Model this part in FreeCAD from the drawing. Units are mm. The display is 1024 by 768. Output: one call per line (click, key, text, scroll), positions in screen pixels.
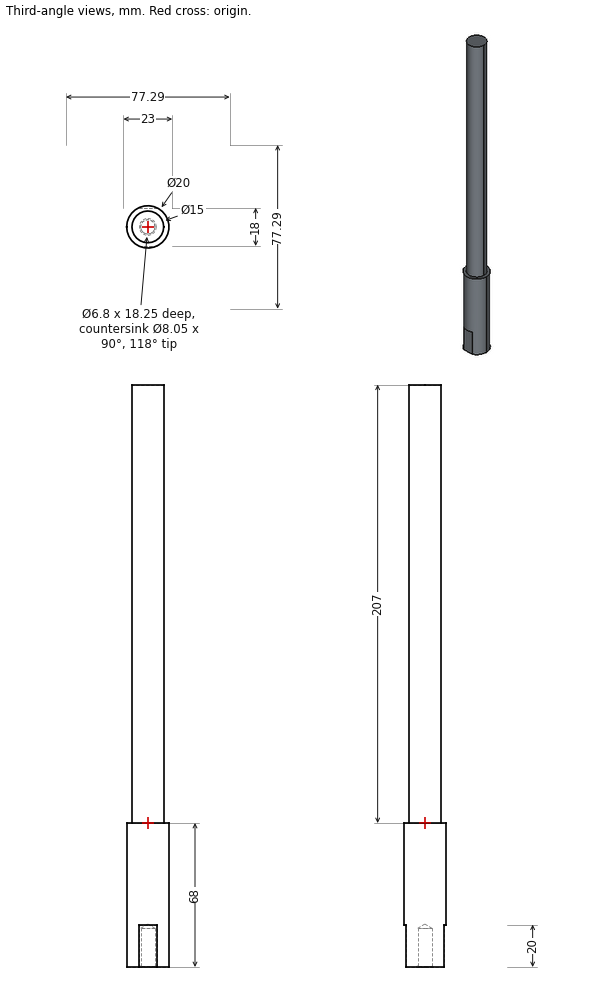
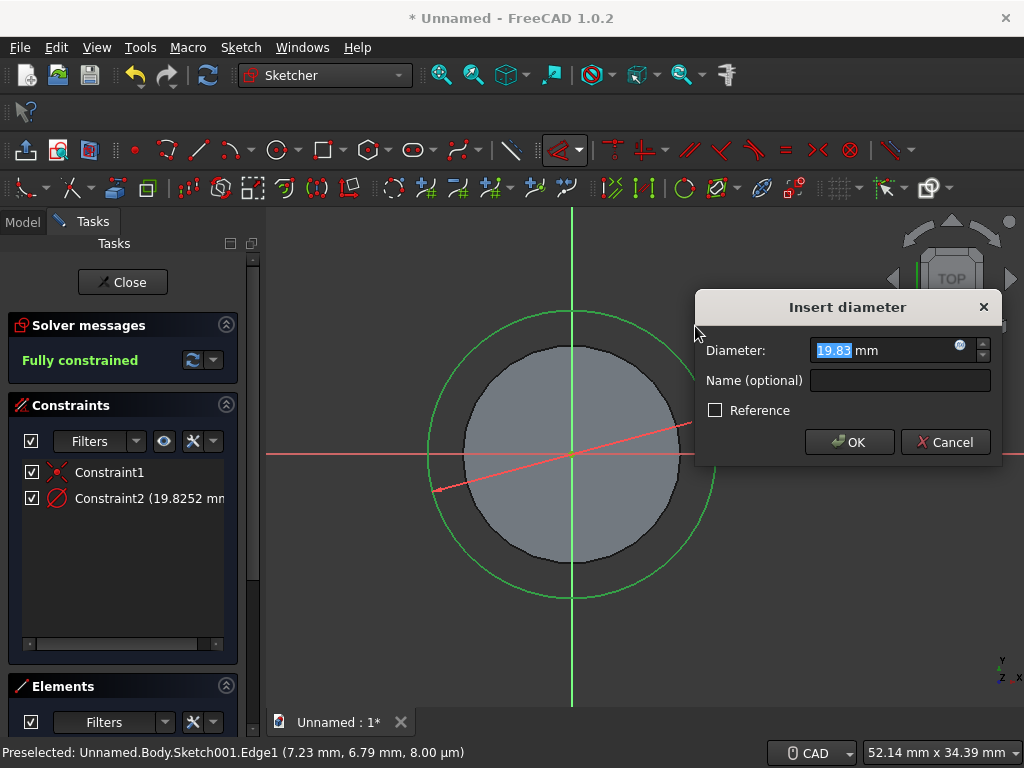
text(20)
key(Return)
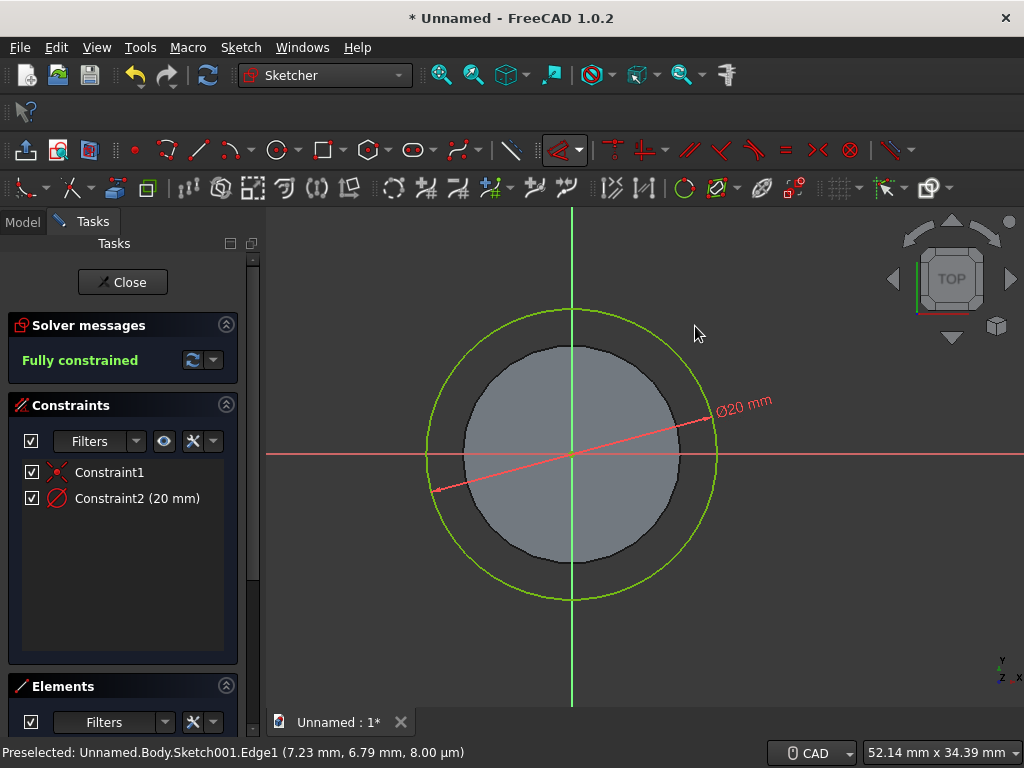
click(123, 282)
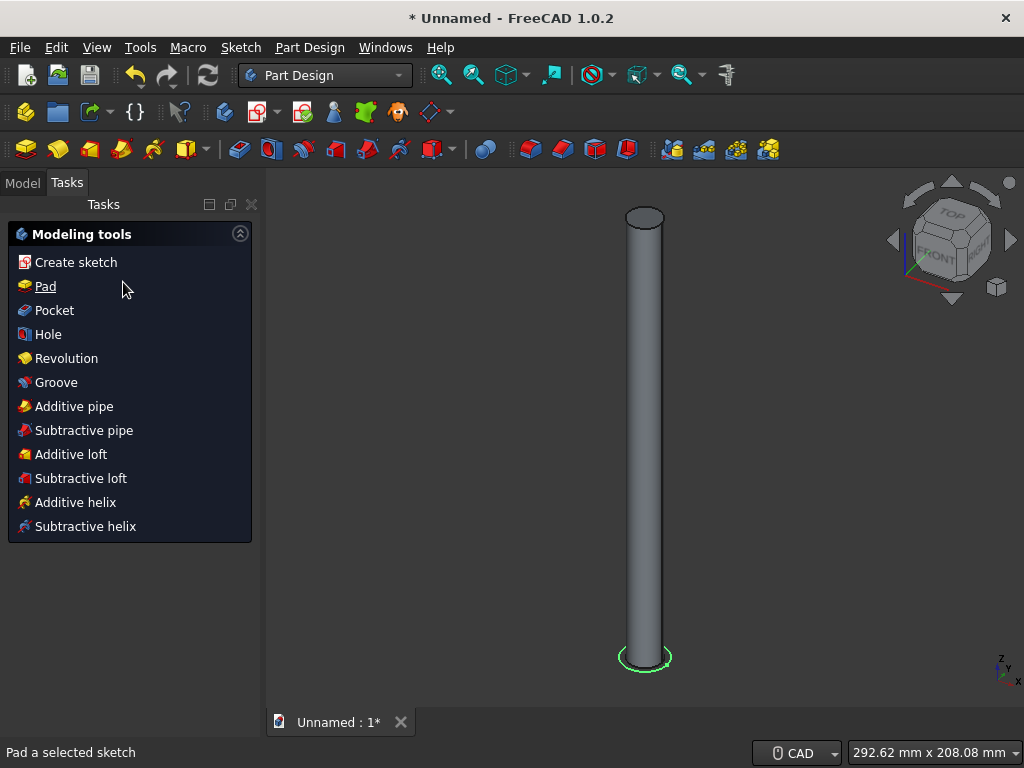
click(26, 150)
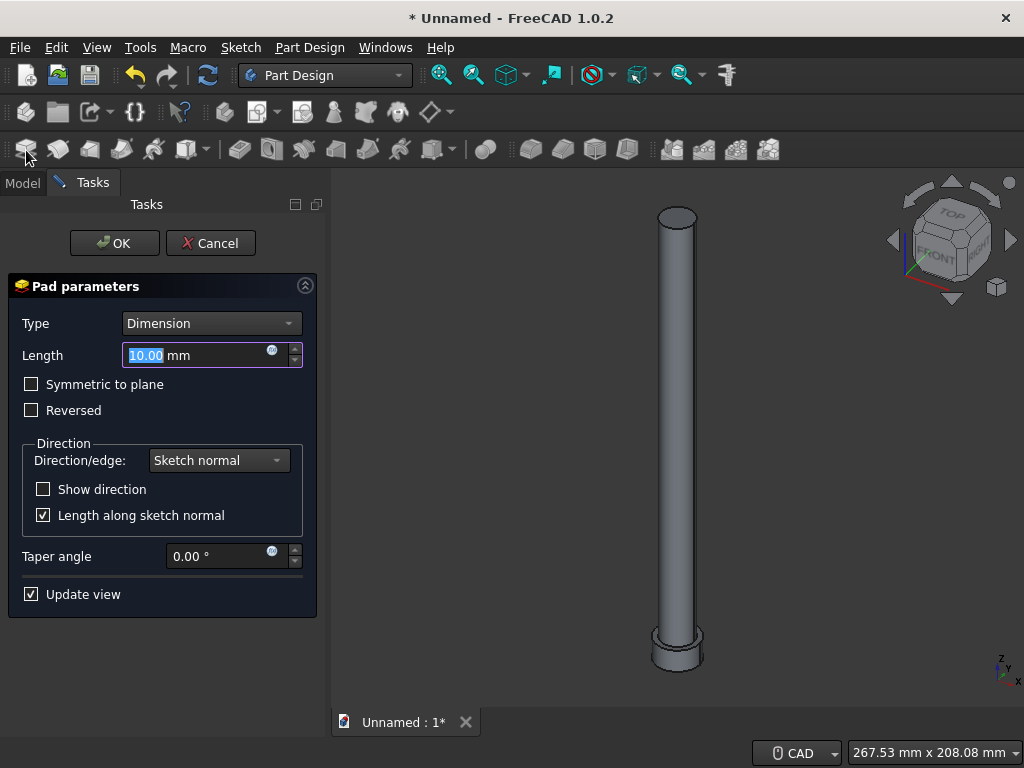
text(68)
key(Tab)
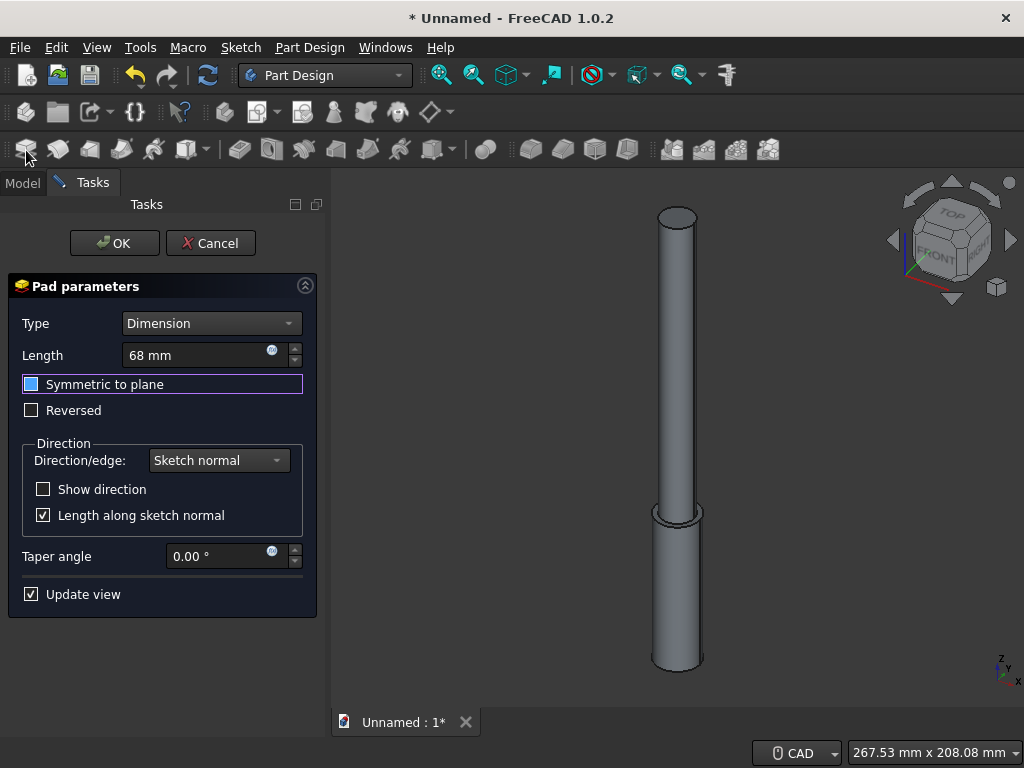
click(30, 410)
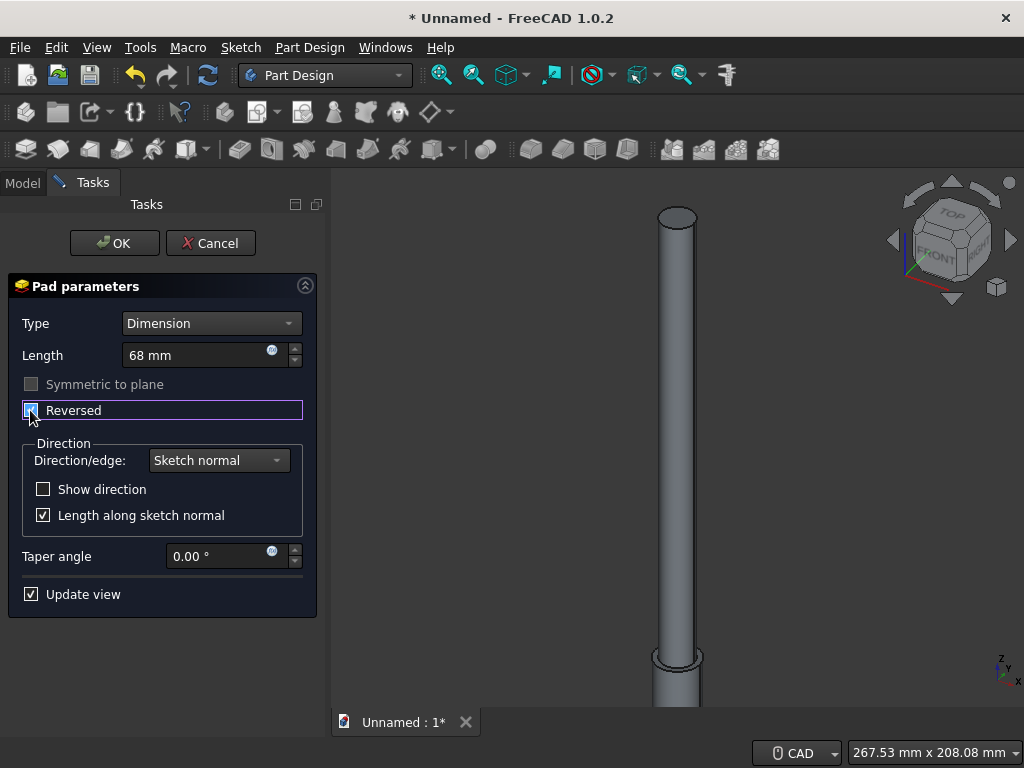
click(115, 243)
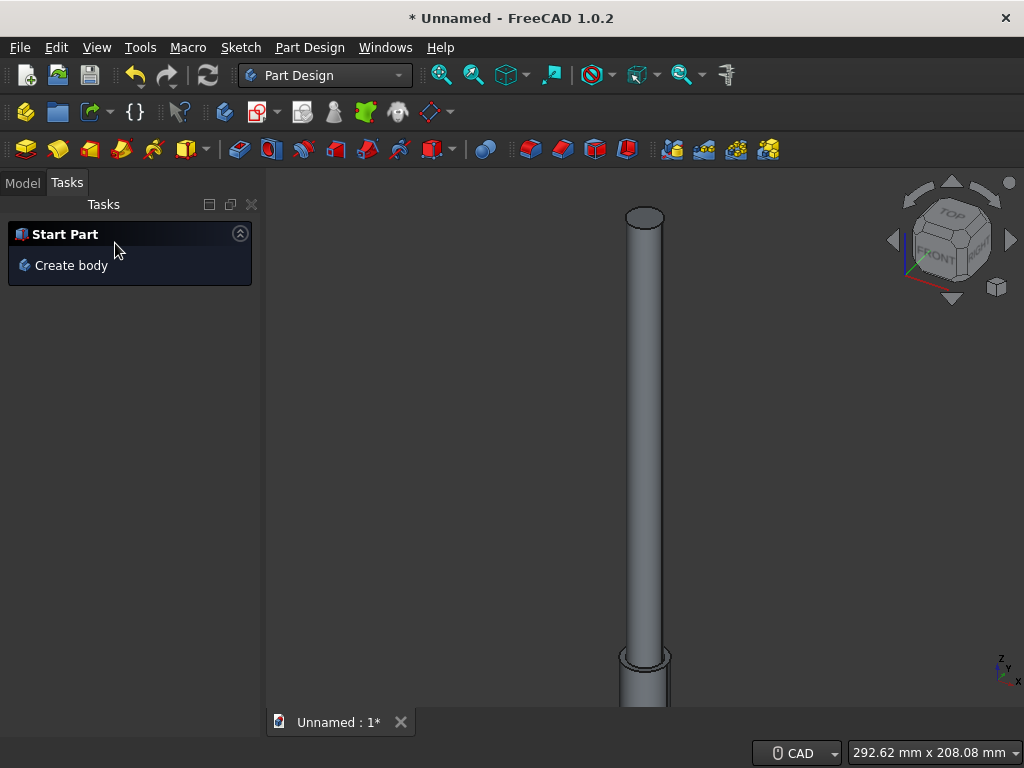
click(442, 76)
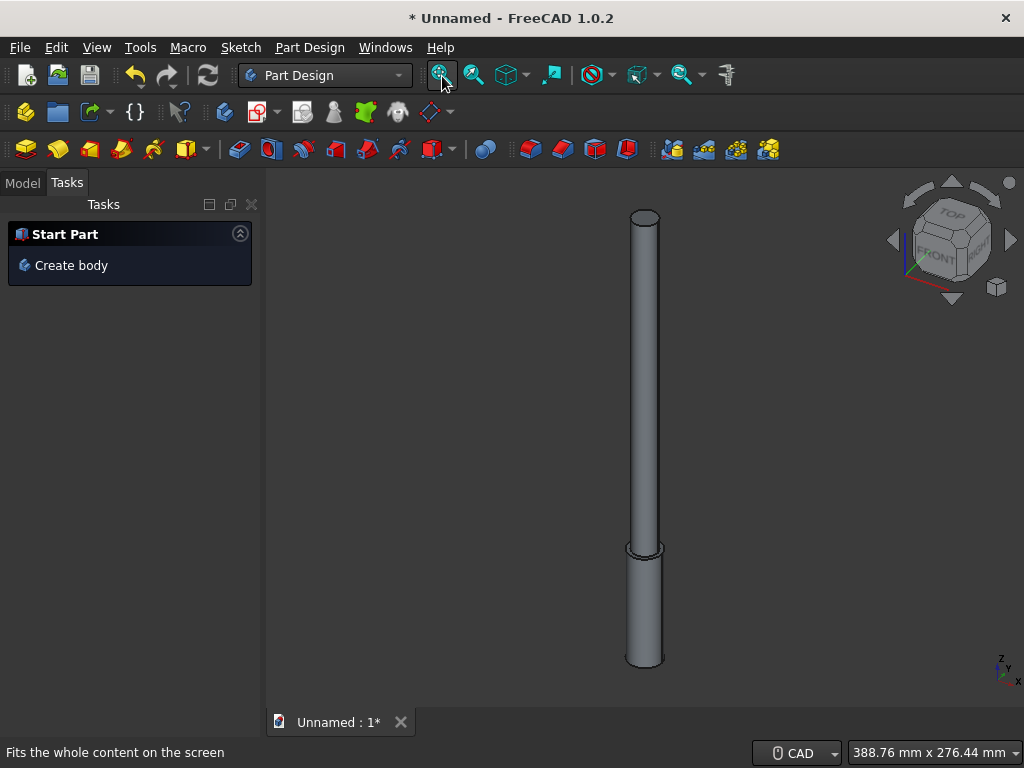
key(5)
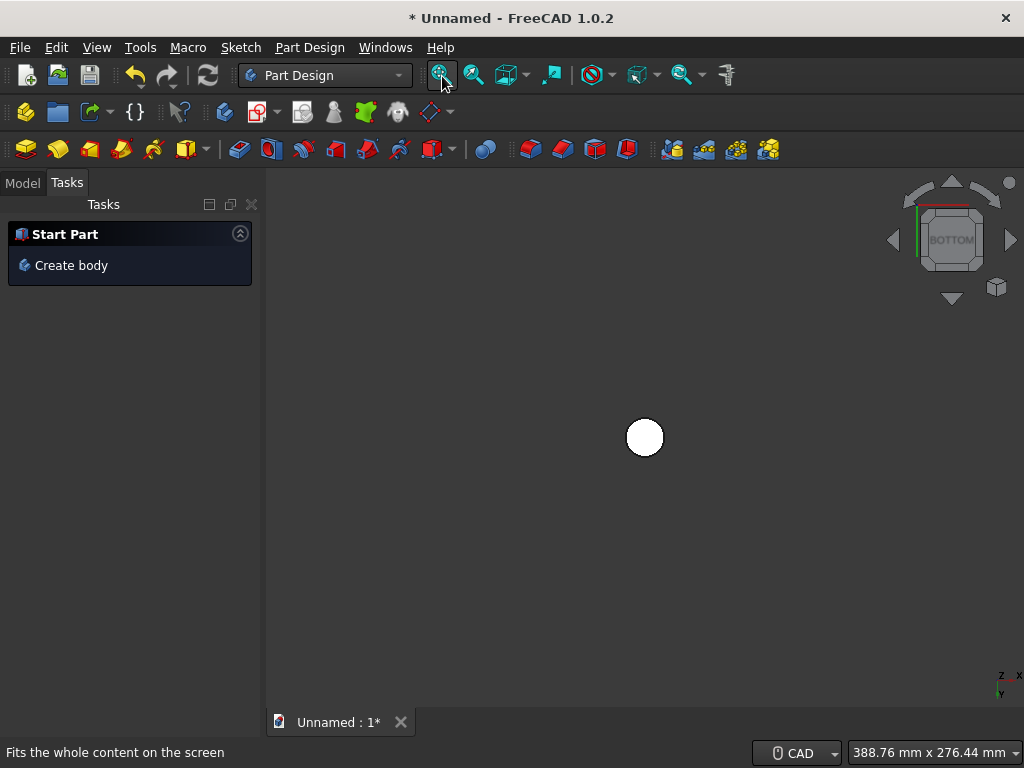
click(442, 76)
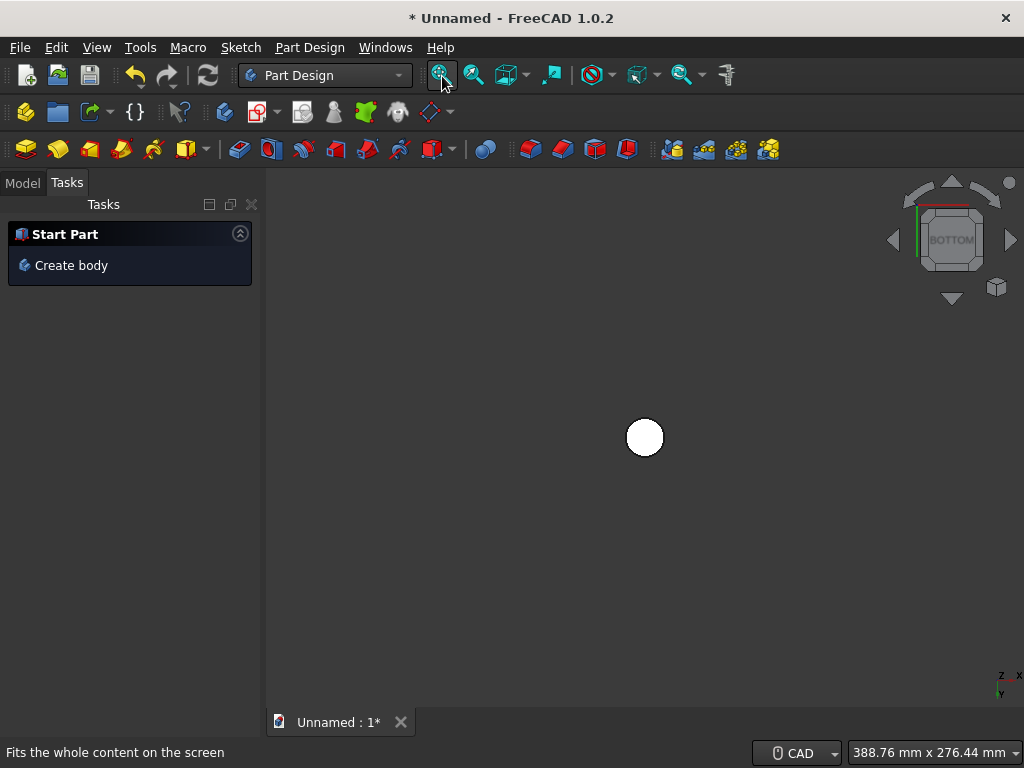
click(645, 436)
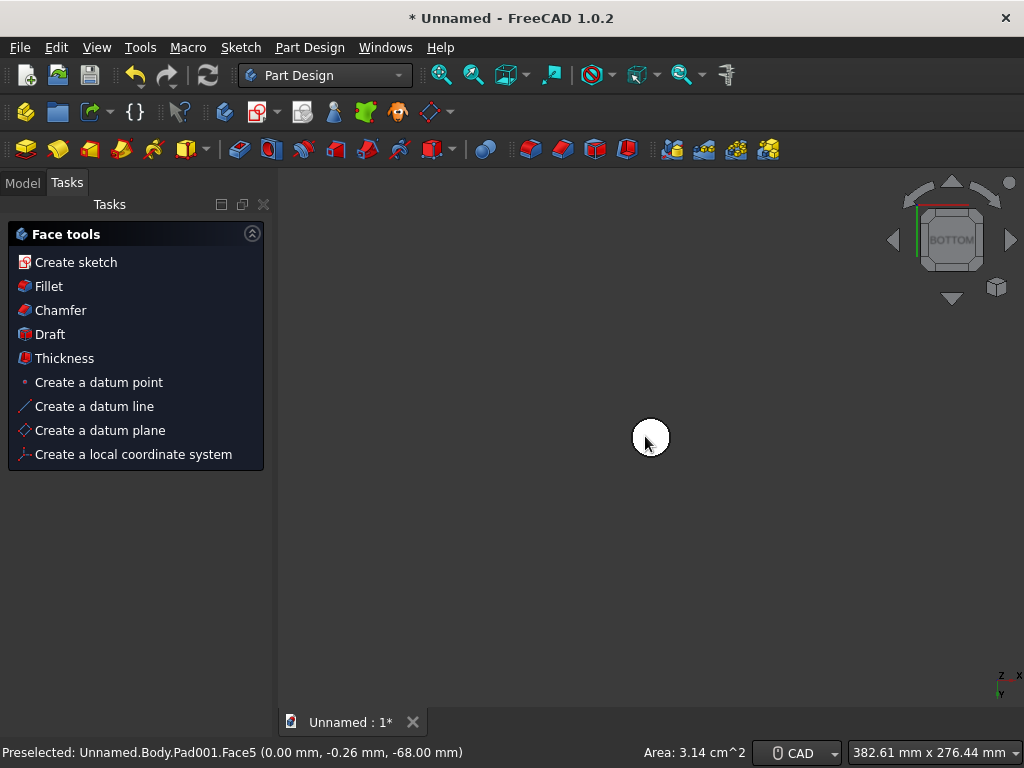
click(258, 112)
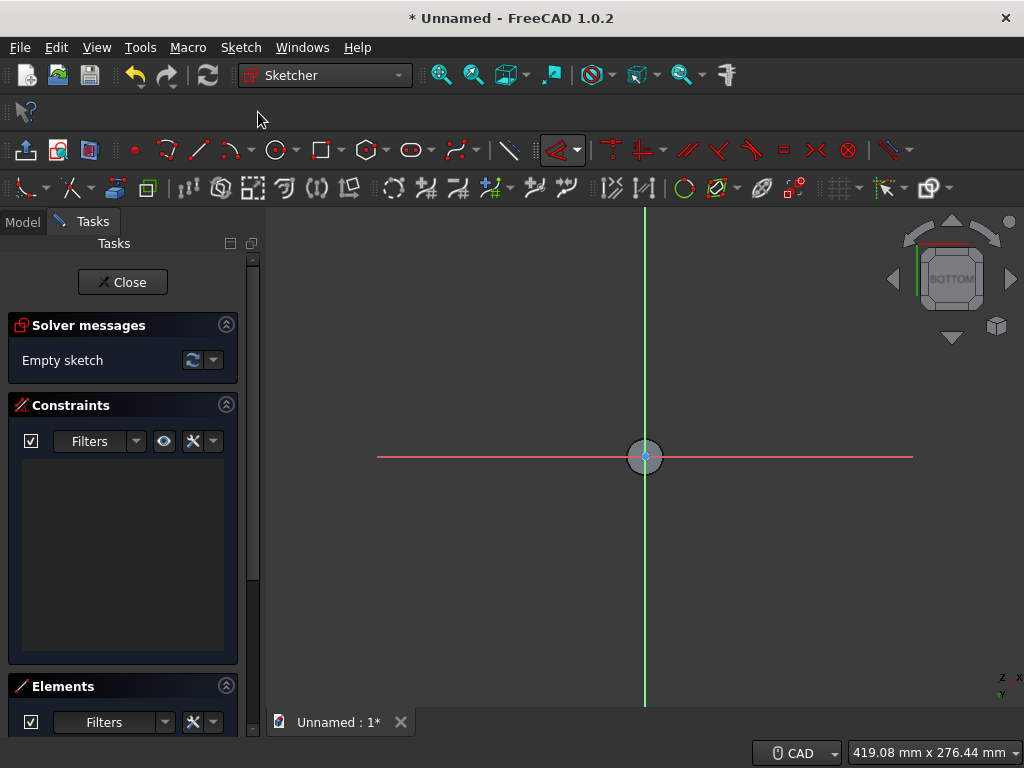
scroll(701, 457, up, 4)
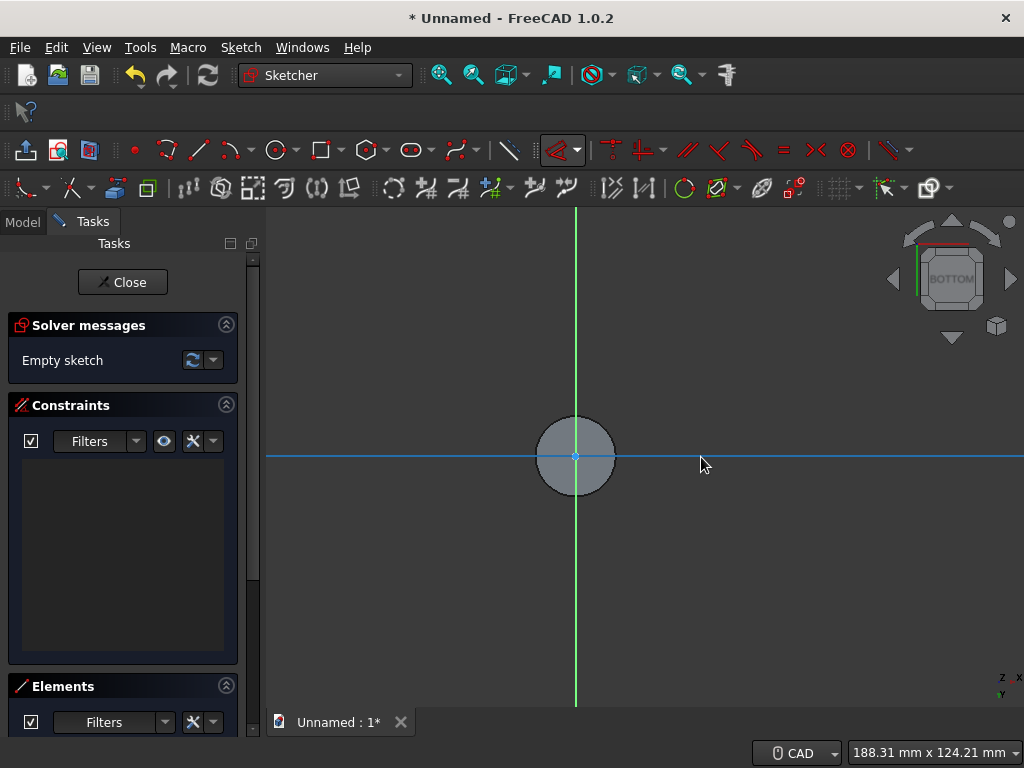
click(344, 150)